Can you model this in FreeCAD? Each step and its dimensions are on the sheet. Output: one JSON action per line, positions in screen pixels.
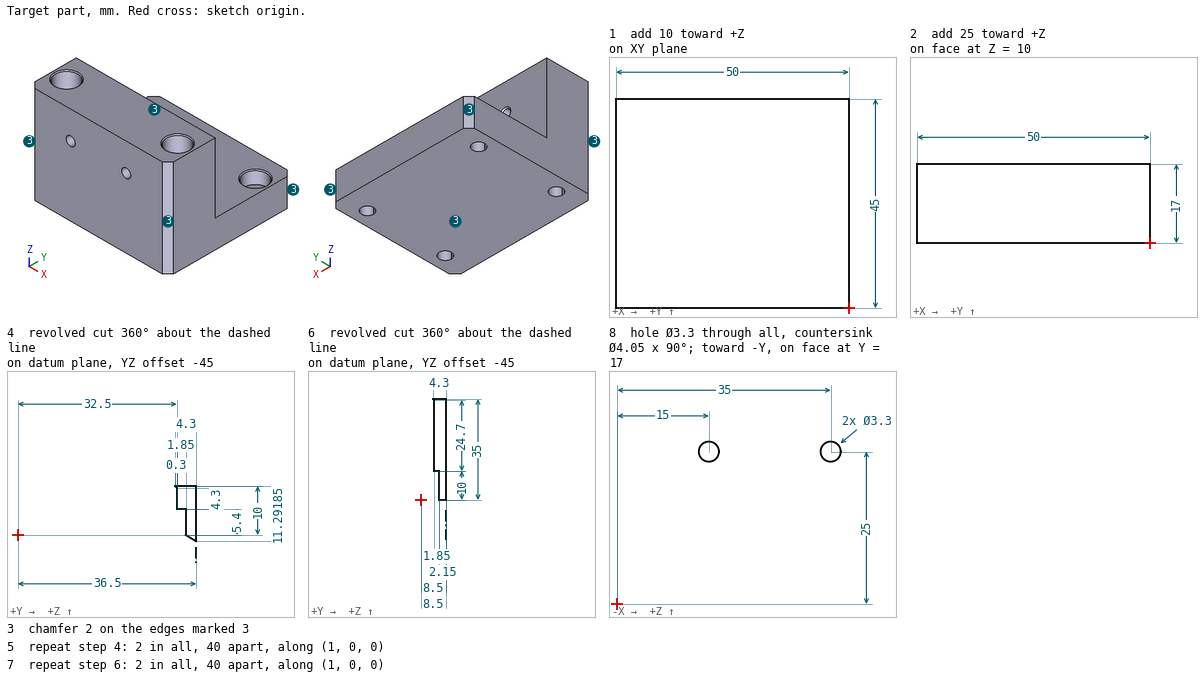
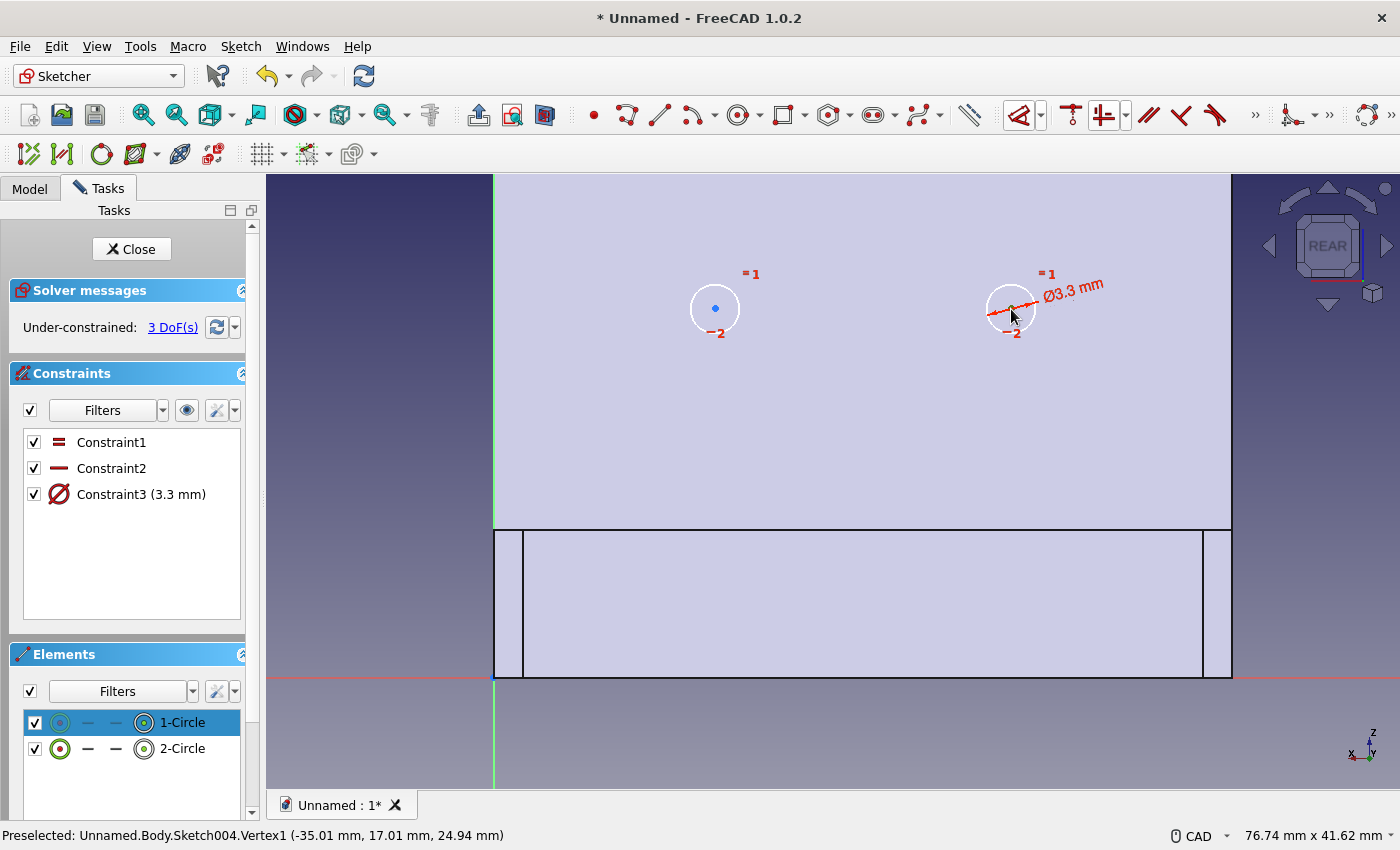
{"action": "key", "text": "l"}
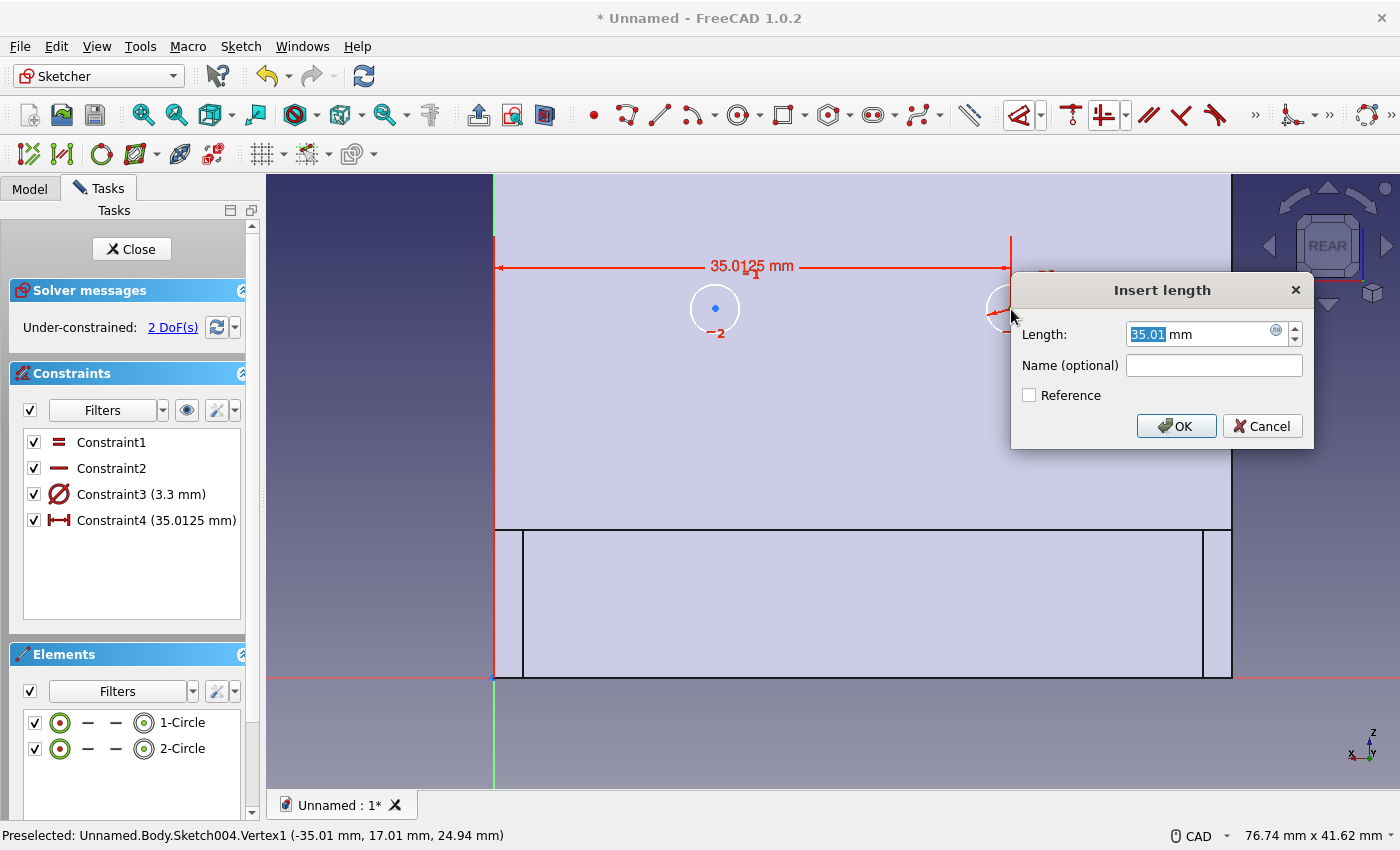
{"action": "type", "text": "35"}
{"action": "key", "text": "Return"}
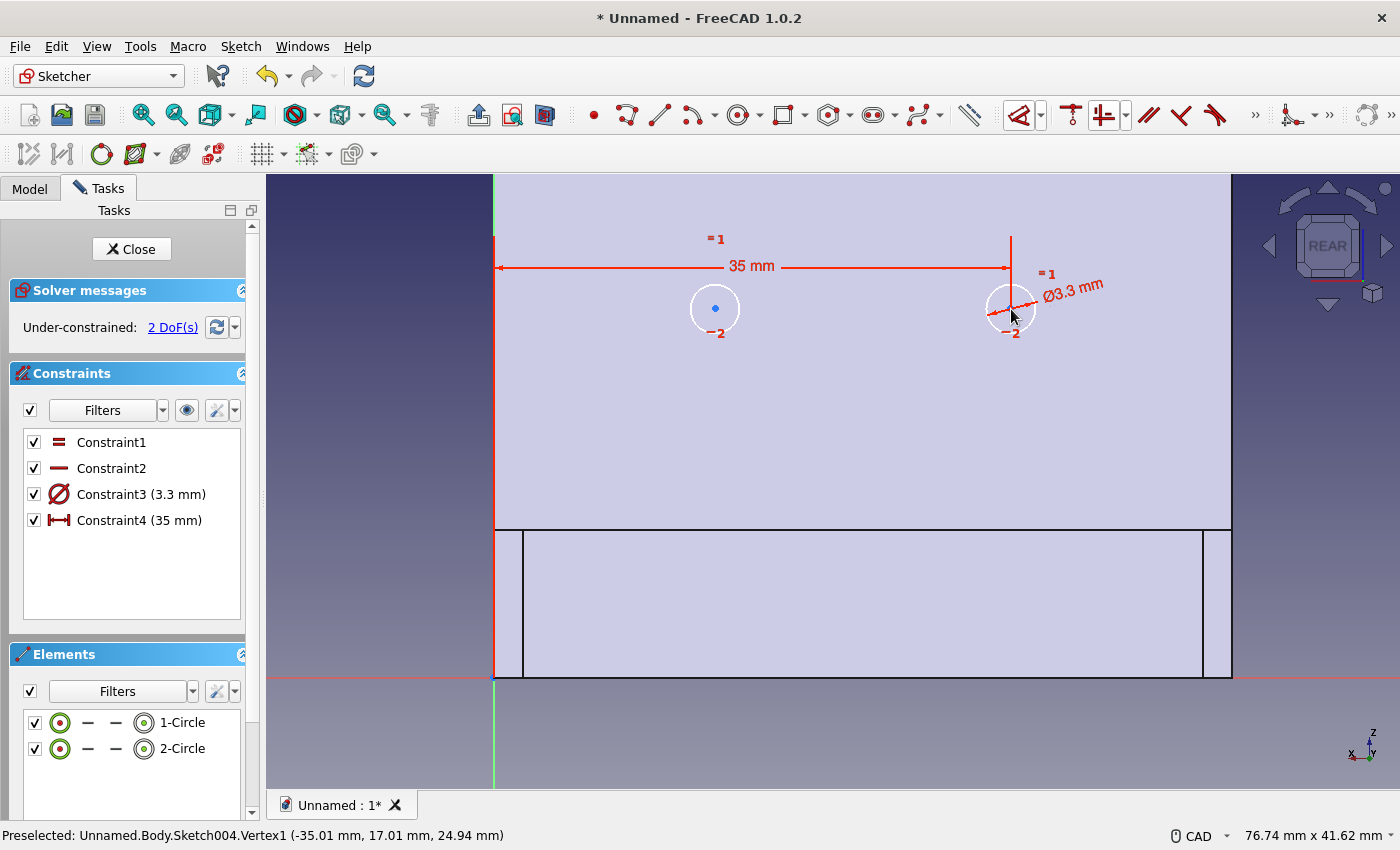
{"action": "left_click", "coordinate": [1011, 309]}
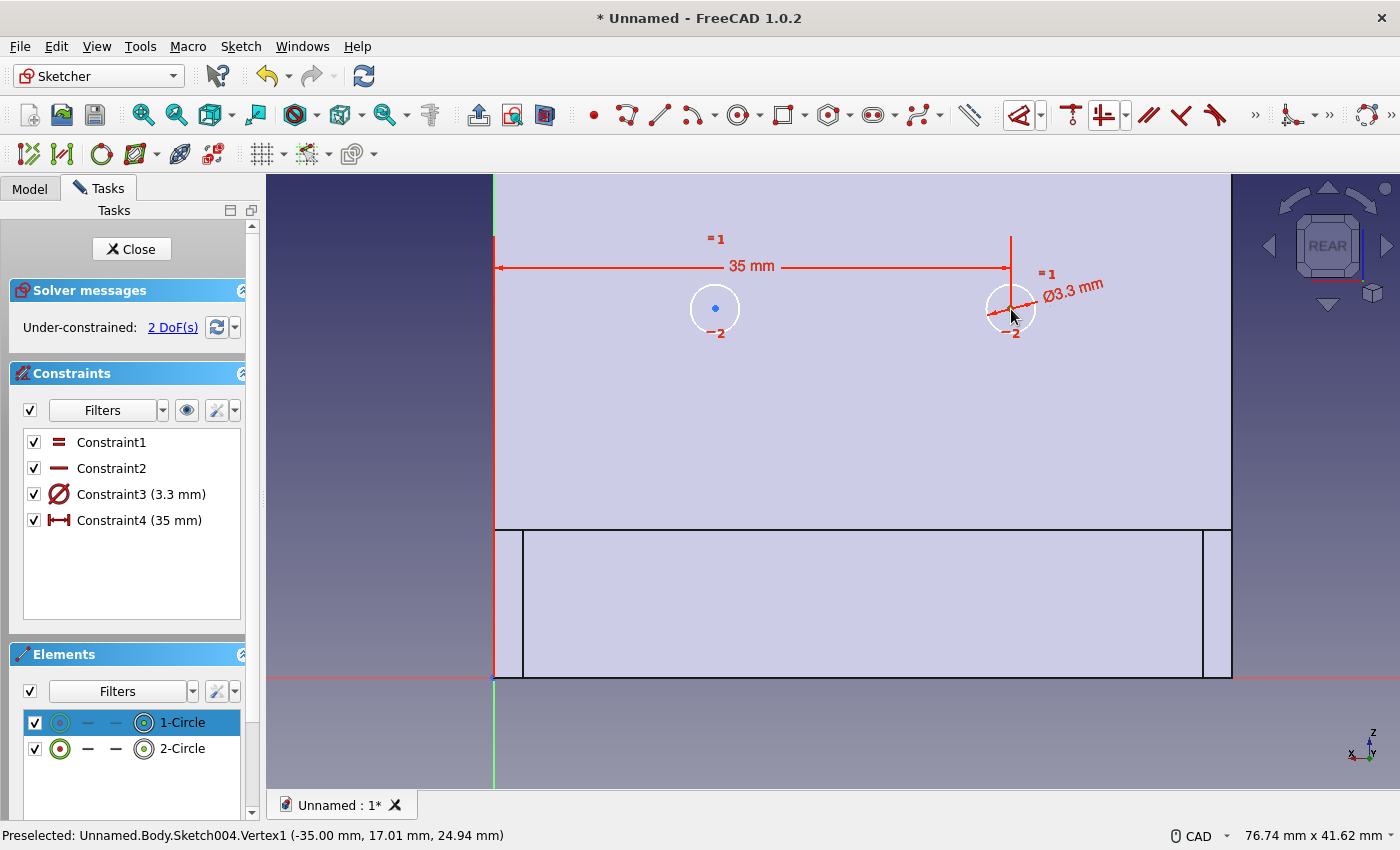
{"action": "left_click", "coordinate": [1040, 116]}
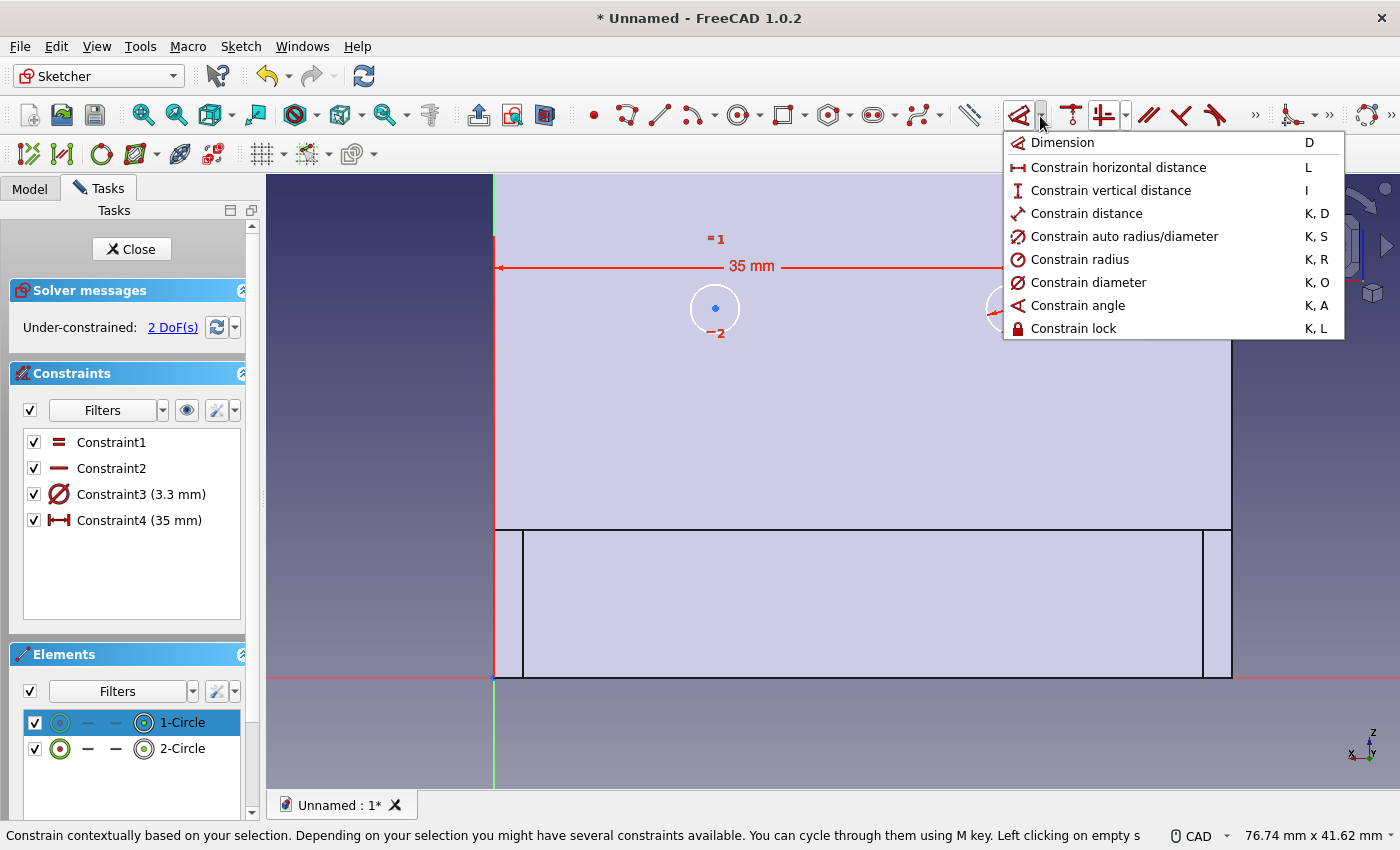
{"action": "left_click", "coordinate": [1174, 190]}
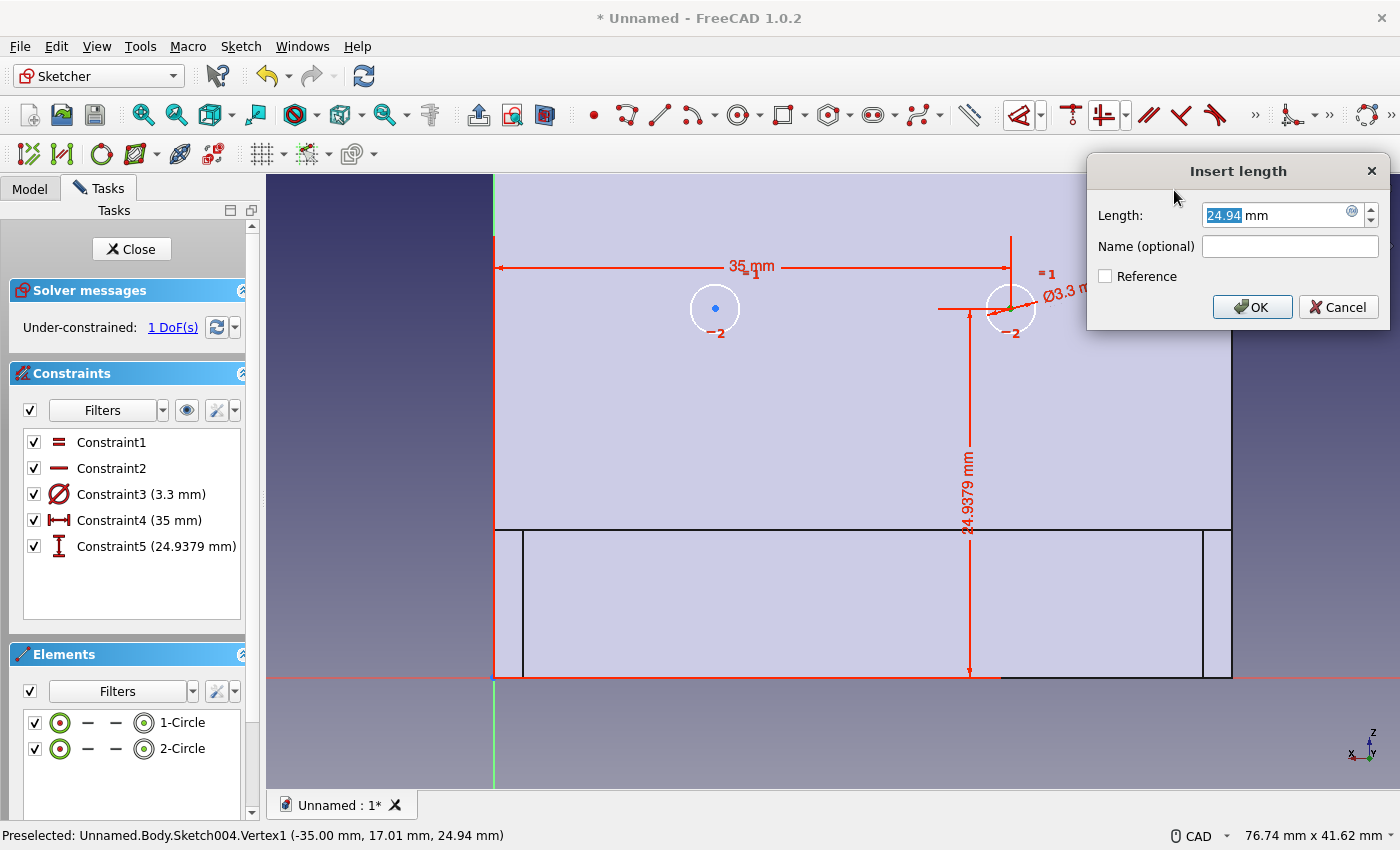
{"action": "type", "text": "25"}
{"action": "key", "text": "Return"}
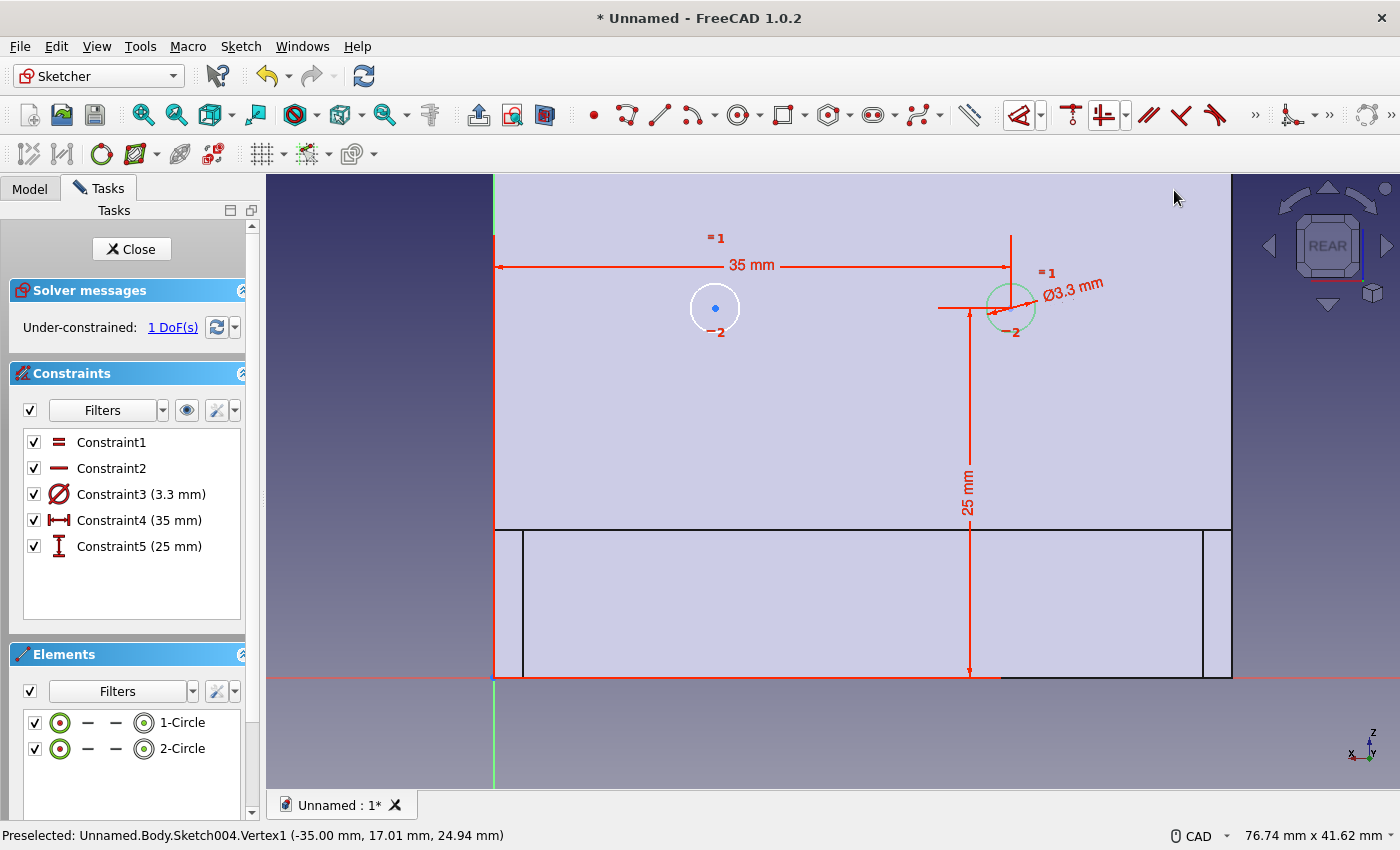
{"action": "left_click", "coordinate": [715, 308]}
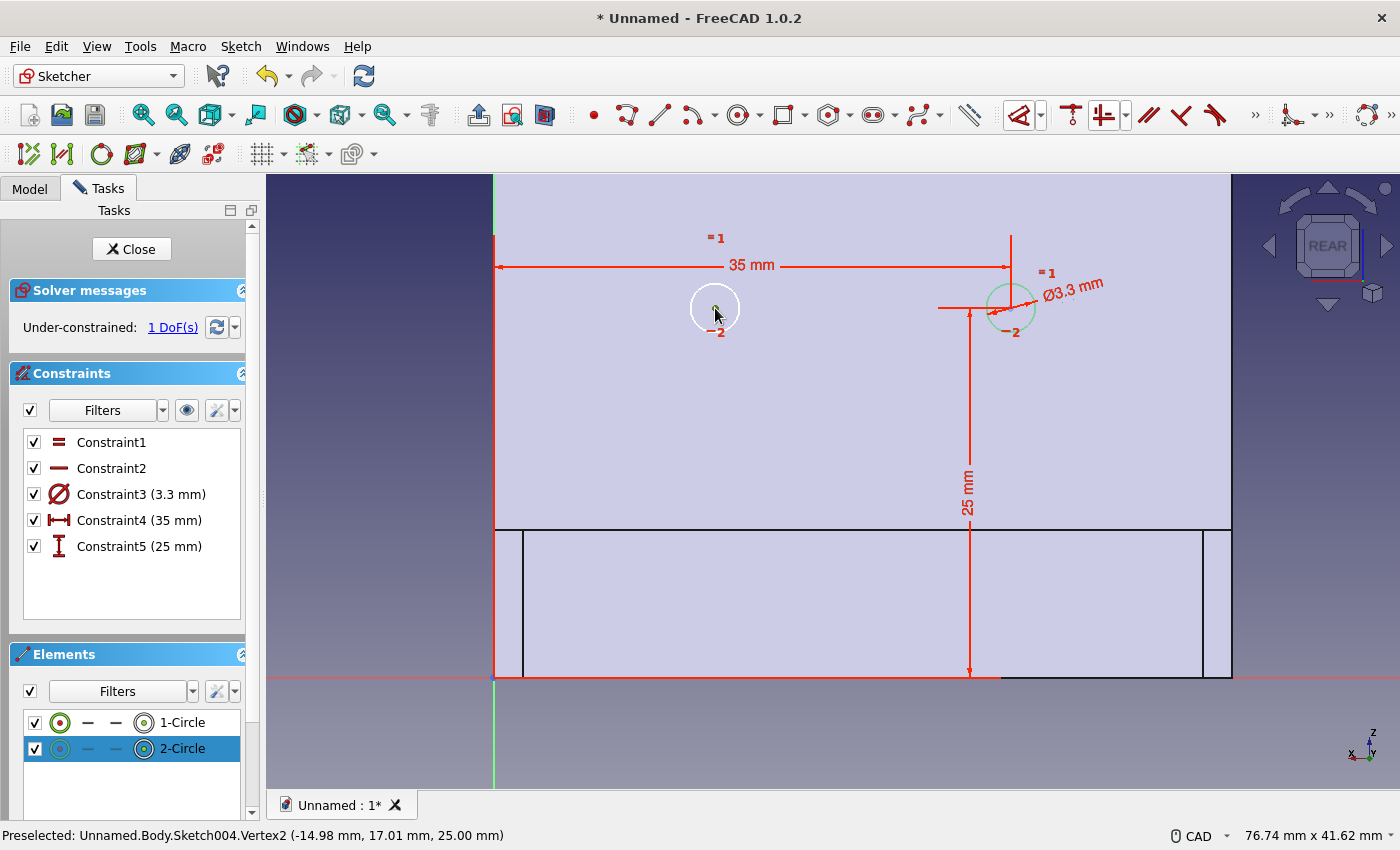
{"action": "left_click", "coordinate": [1040, 116]}